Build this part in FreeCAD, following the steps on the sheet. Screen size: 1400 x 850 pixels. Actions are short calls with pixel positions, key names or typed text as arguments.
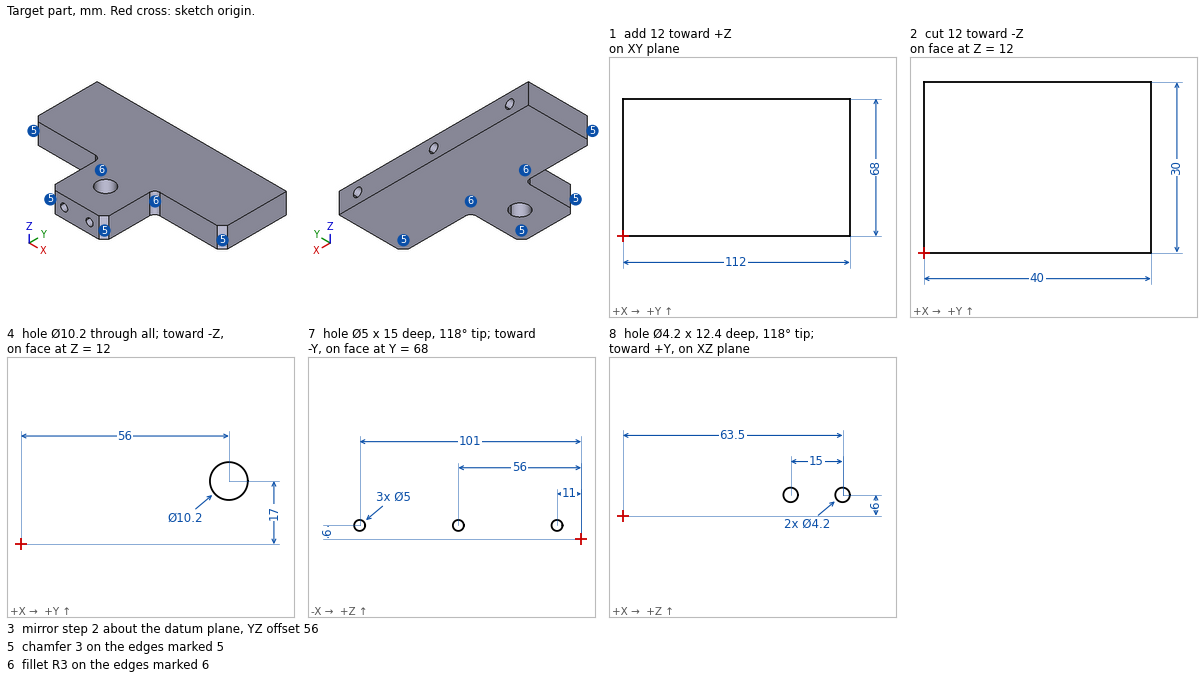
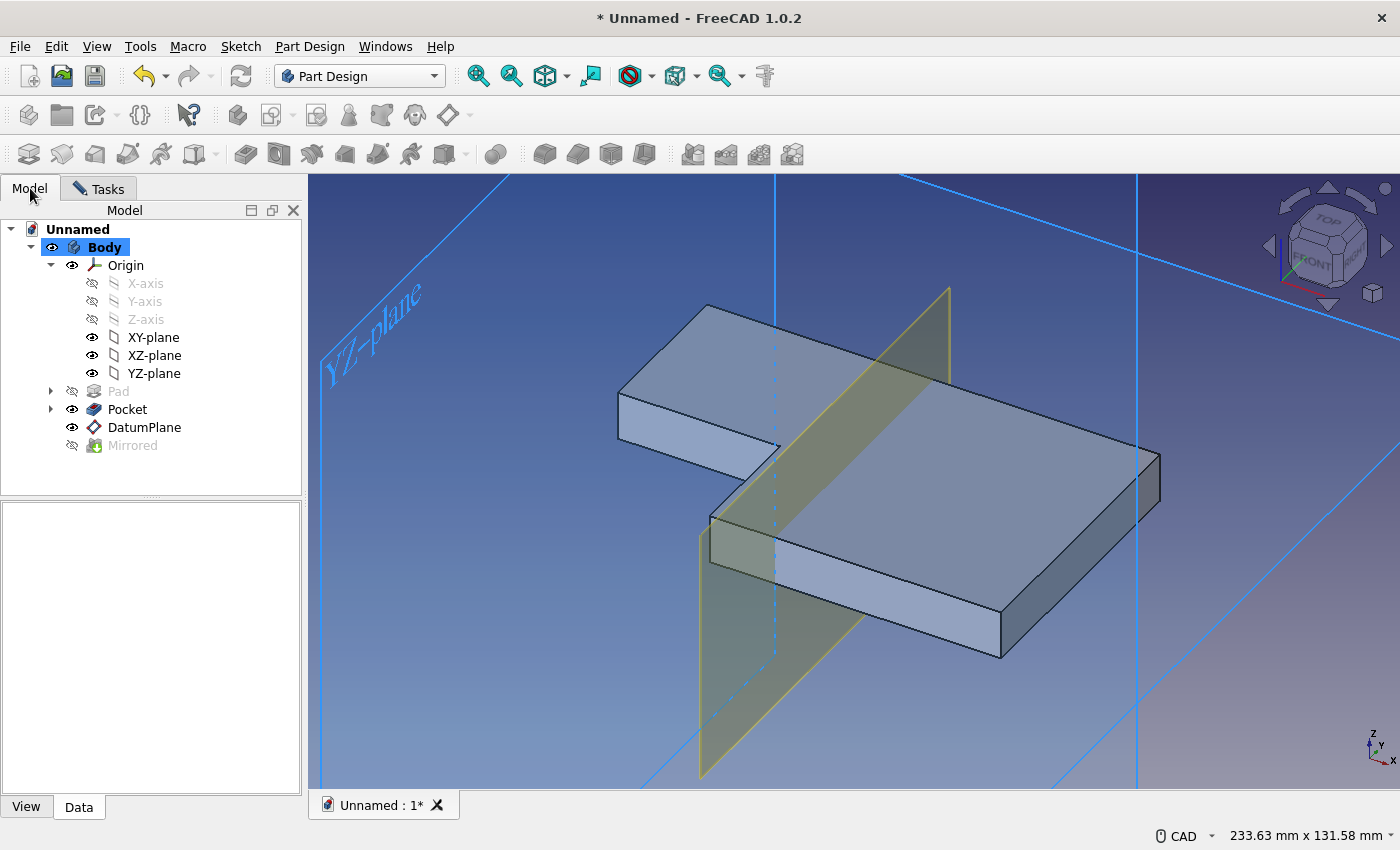
click(117, 427)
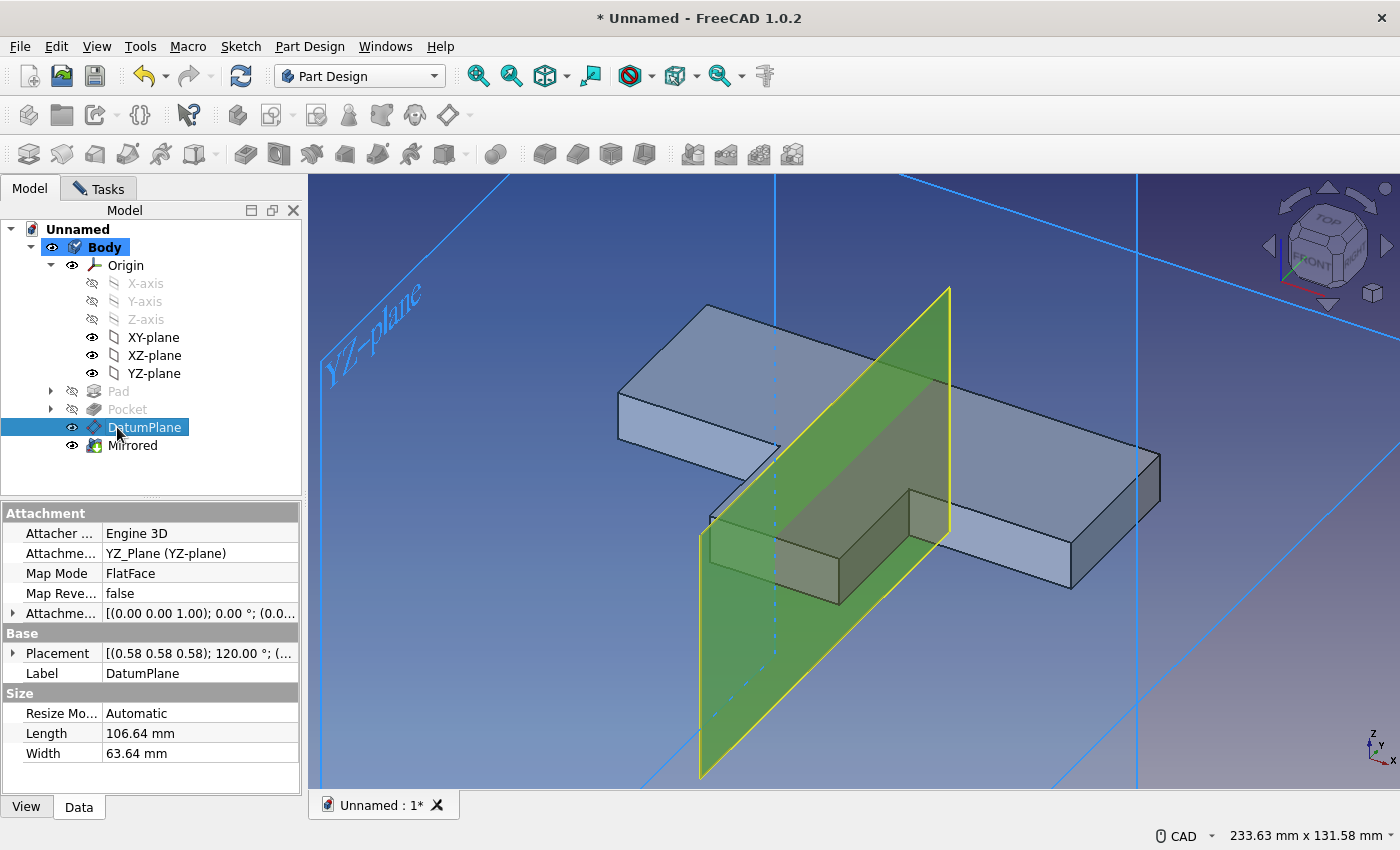
click(98, 188)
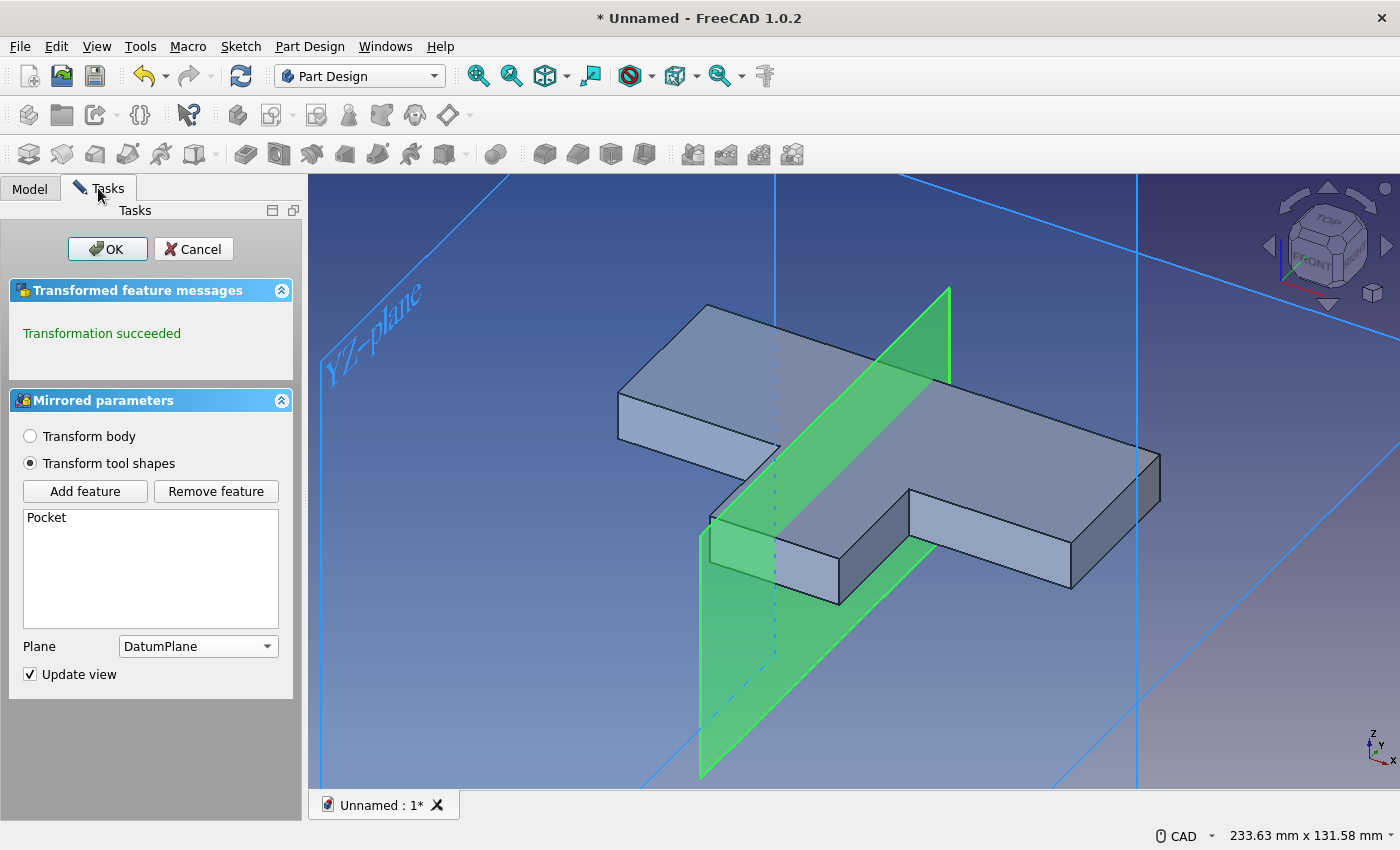
click(108, 249)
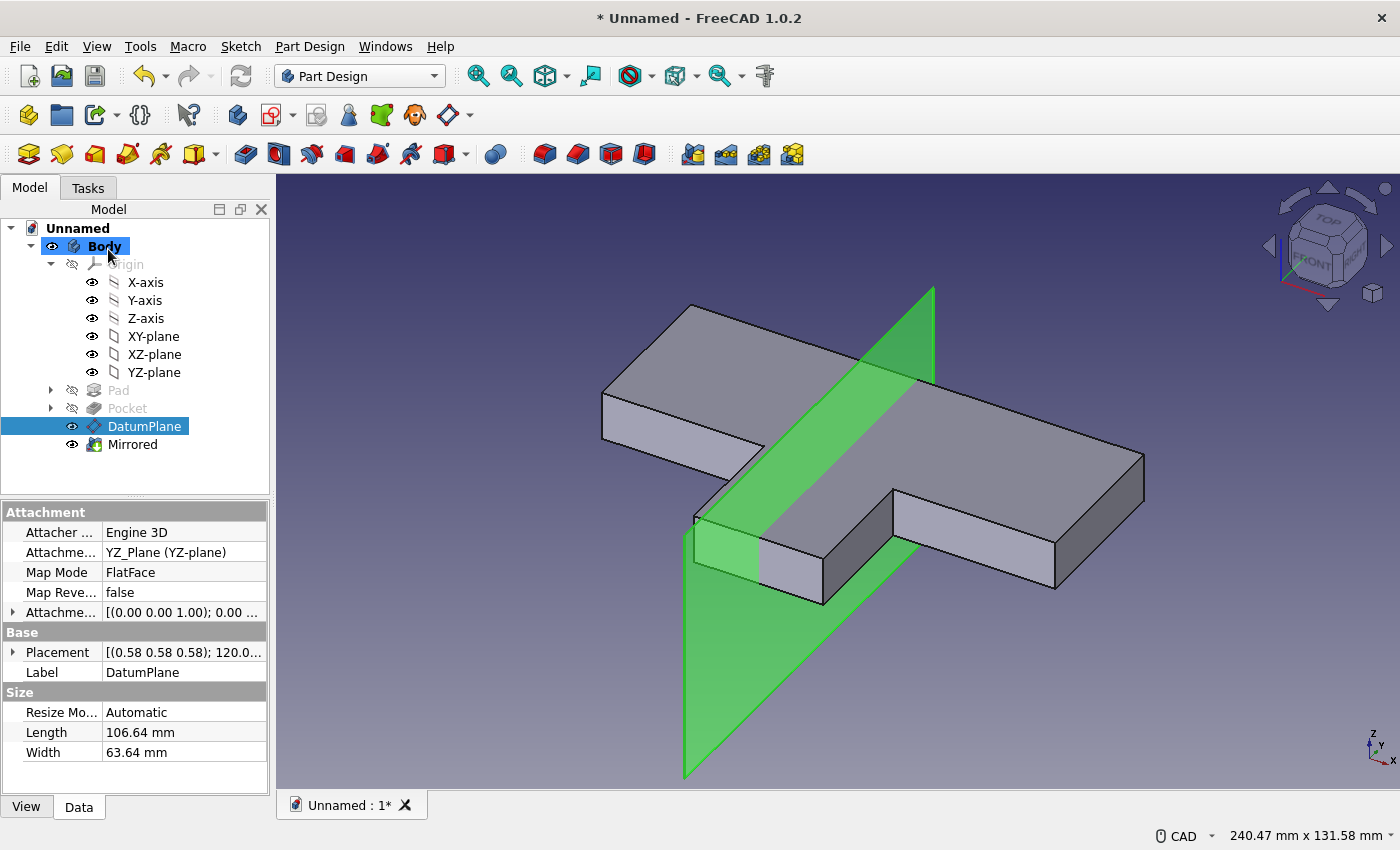
click(117, 426)
key(space)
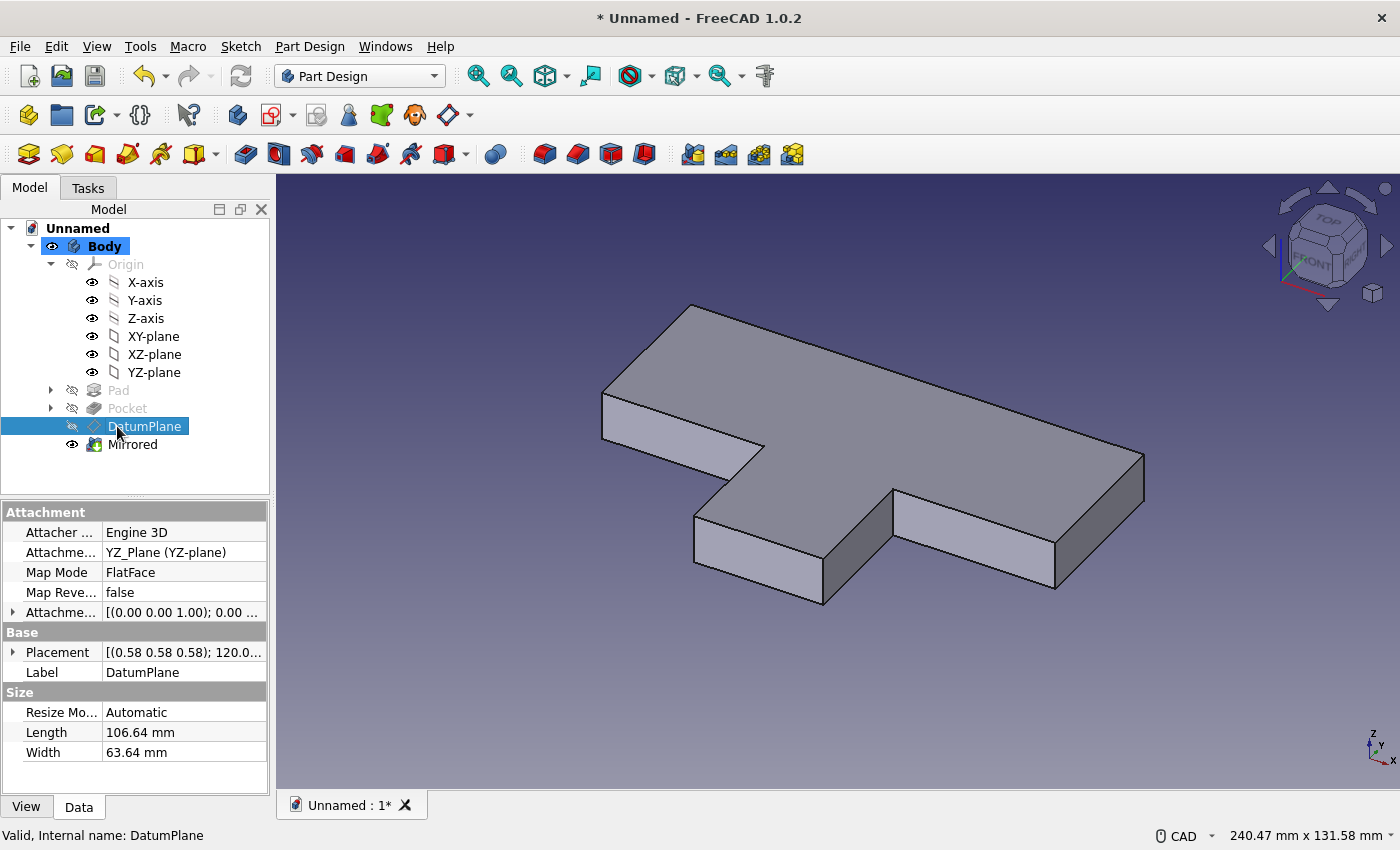
click(861, 435)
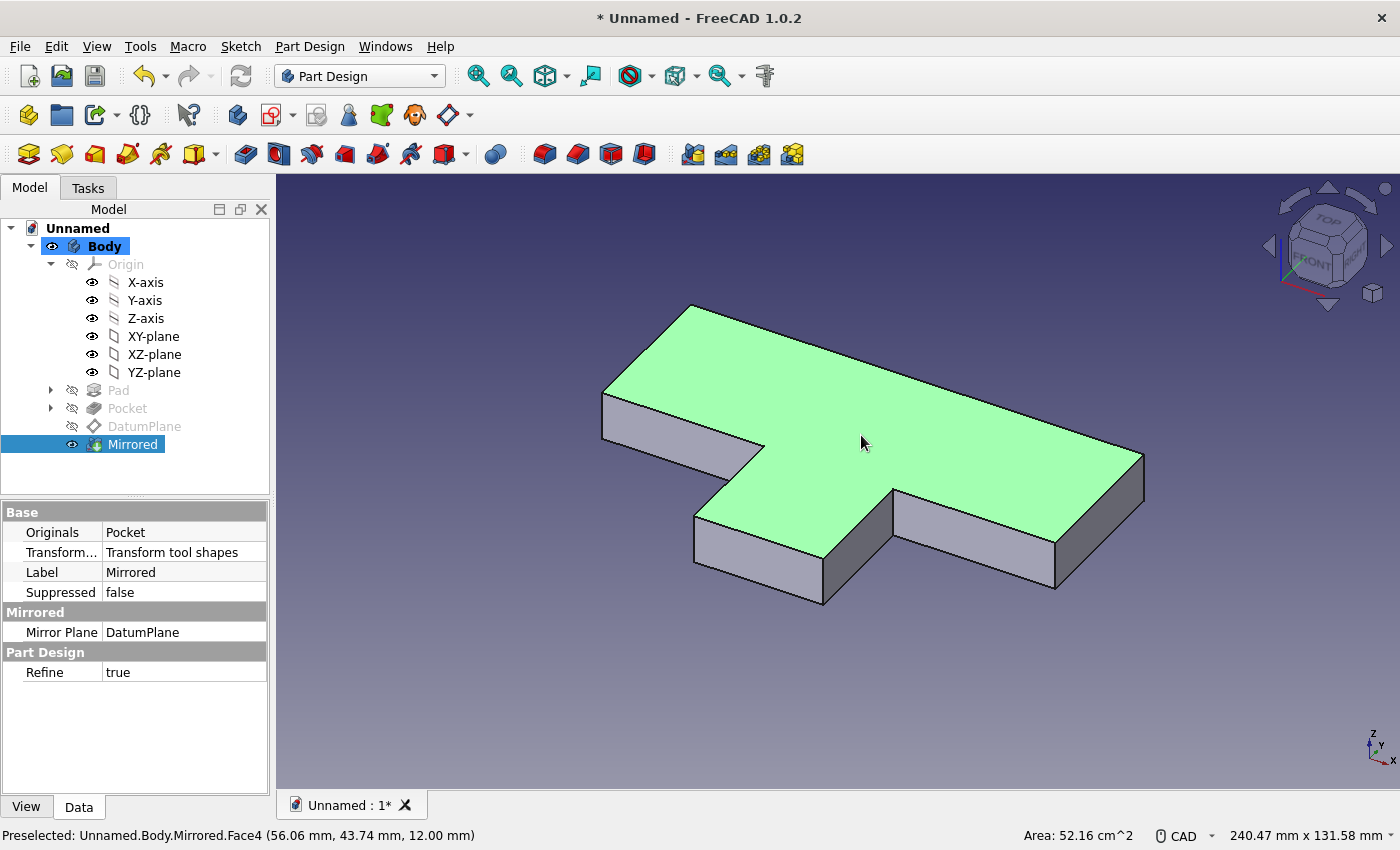
click(270, 116)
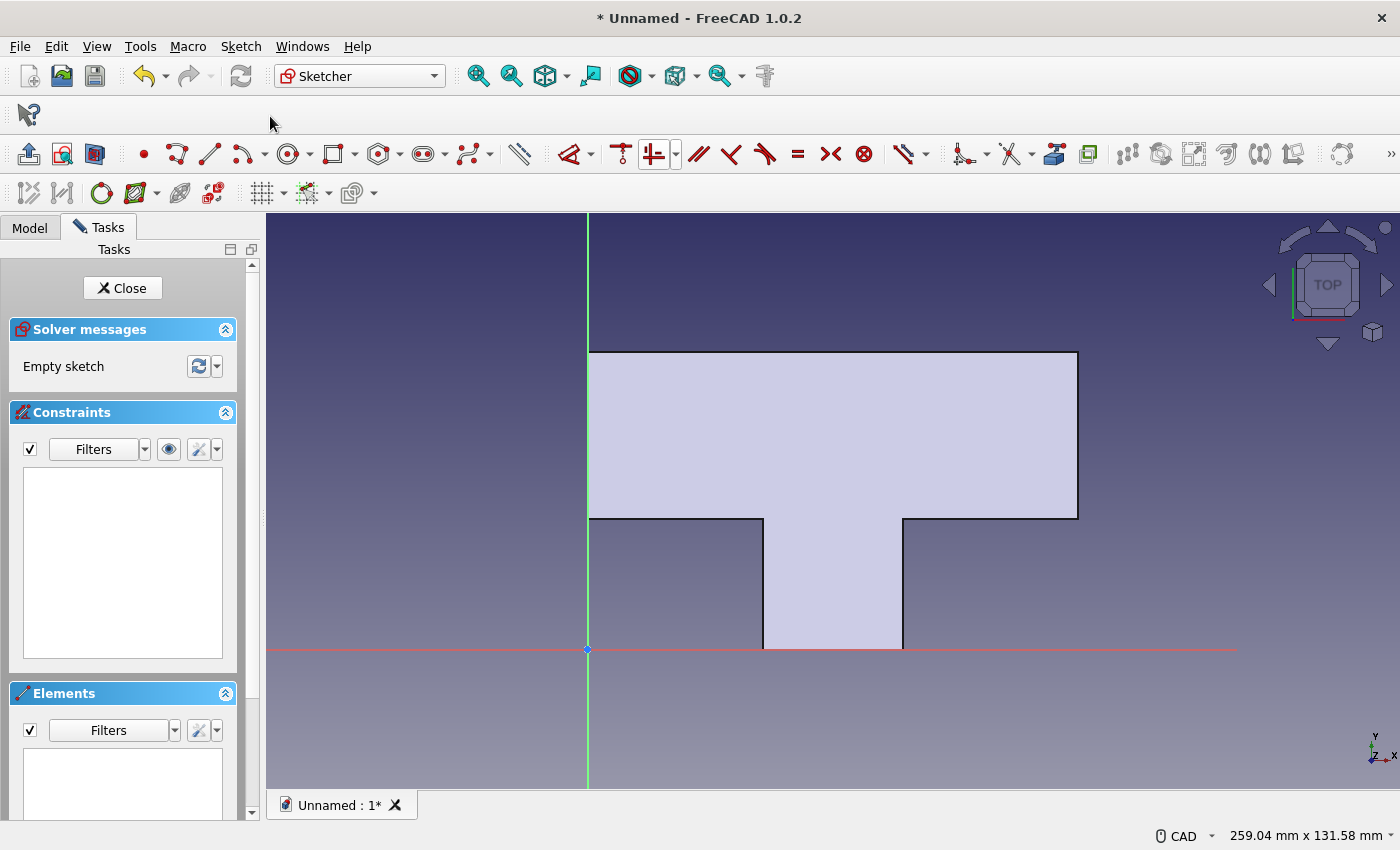
scroll(842, 585, up, 11)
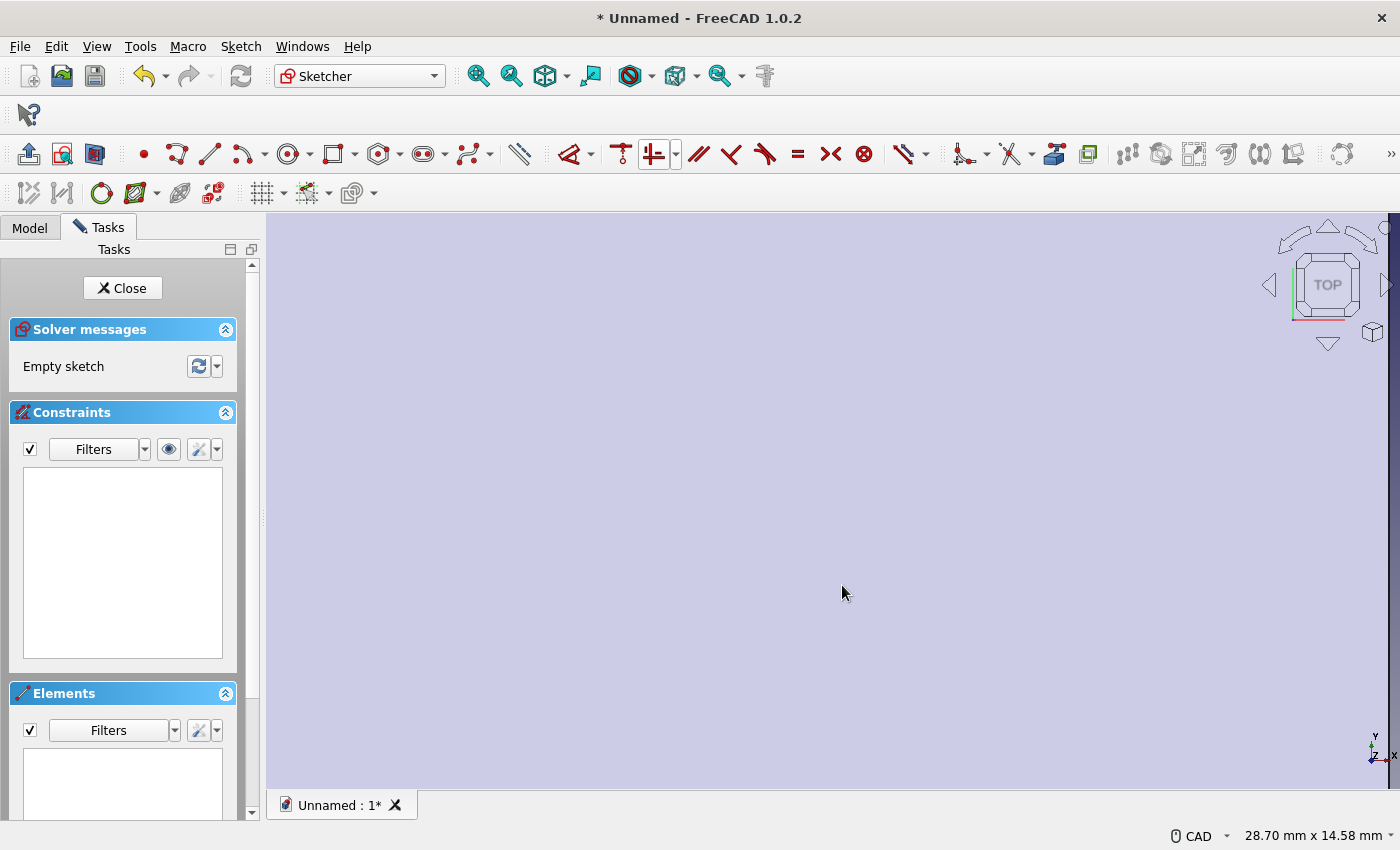
key(g)
key(c)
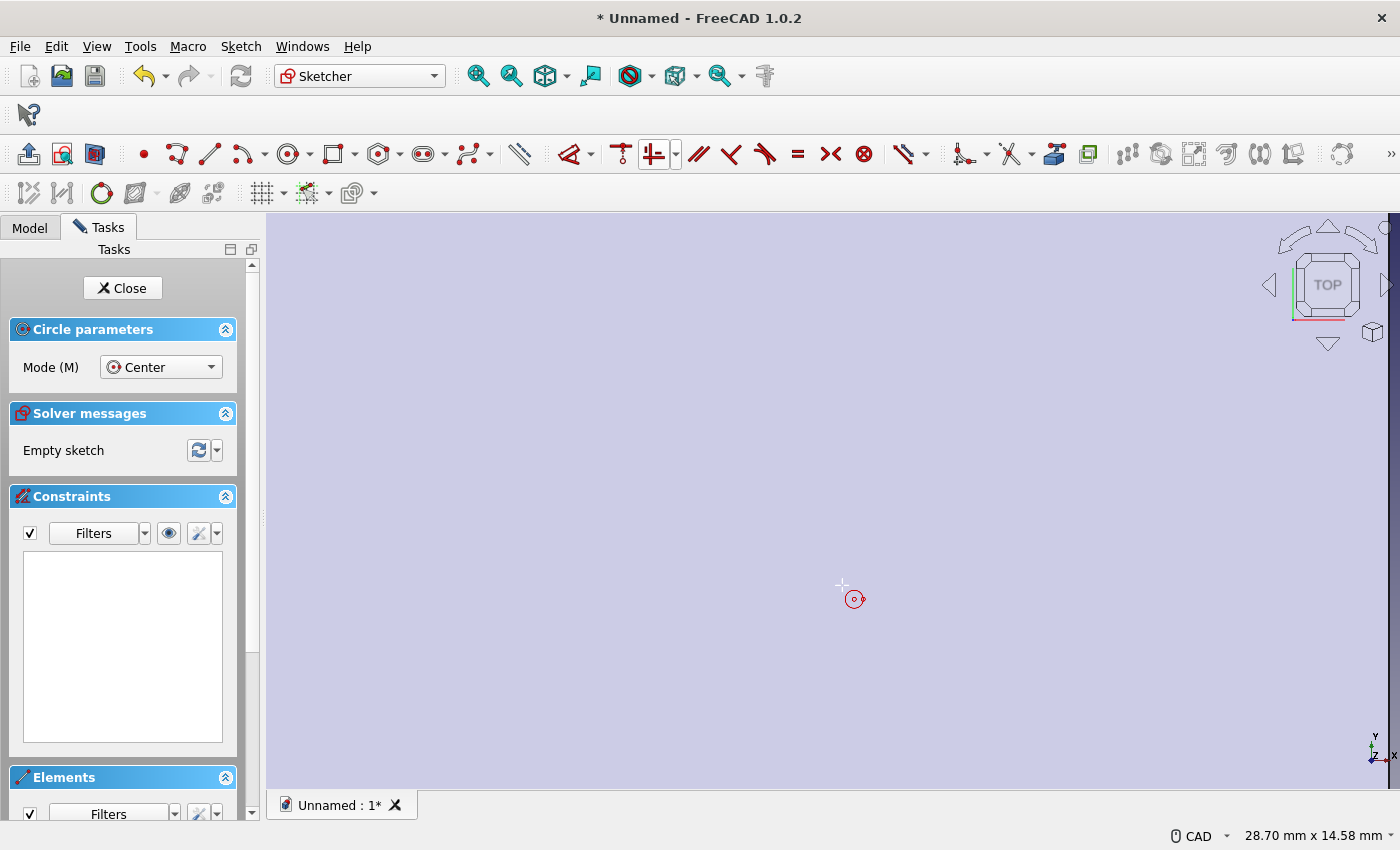
click(757, 493)
click(899, 351)
key(Escape)